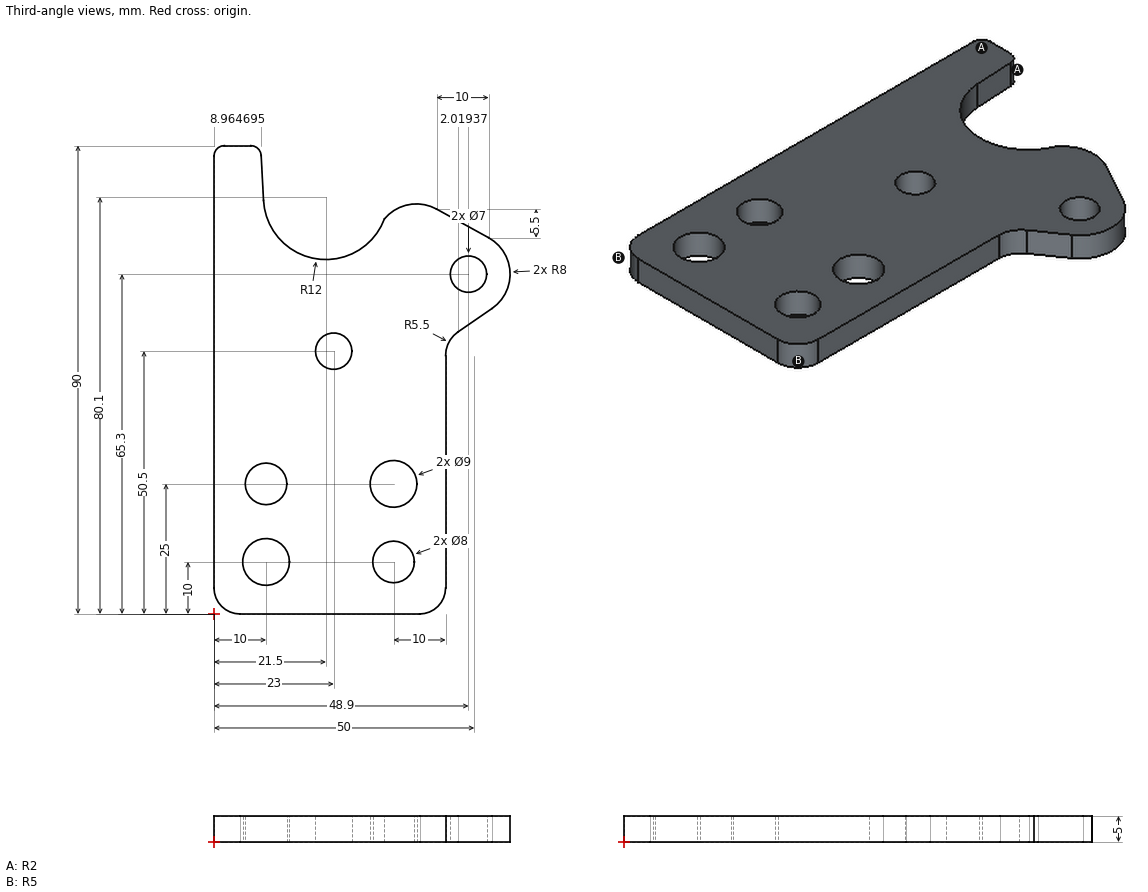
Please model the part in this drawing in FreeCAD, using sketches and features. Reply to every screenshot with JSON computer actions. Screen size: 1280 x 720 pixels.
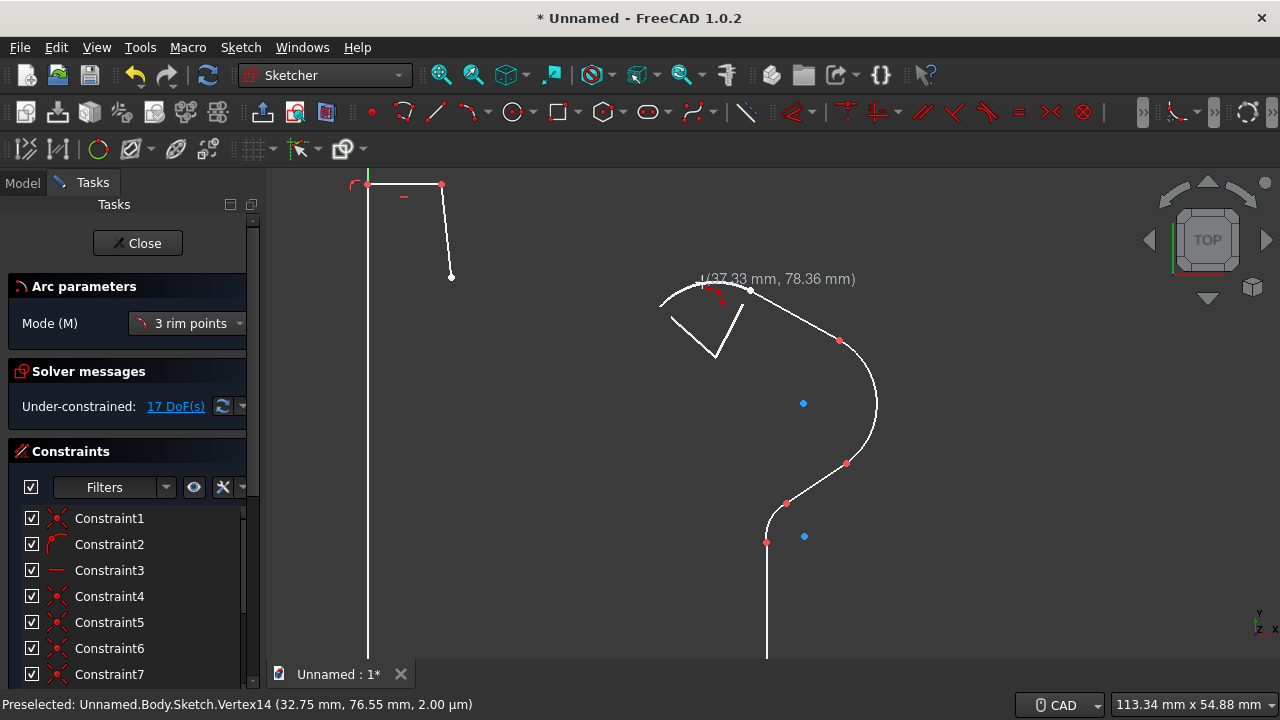
{"action": "left_click", "coordinate": [702, 281]}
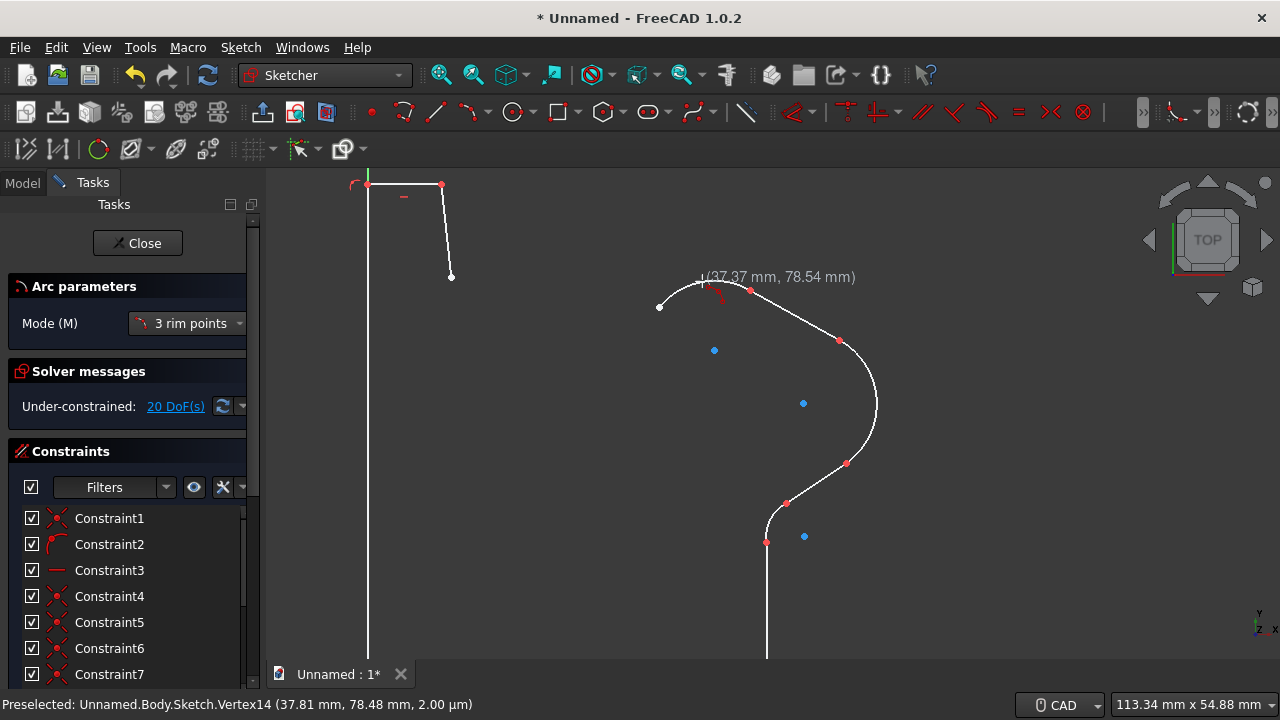
{"action": "left_click", "coordinate": [660, 307]}
{"action": "left_click", "coordinate": [451, 277]}
{"action": "left_click", "coordinate": [544, 374]}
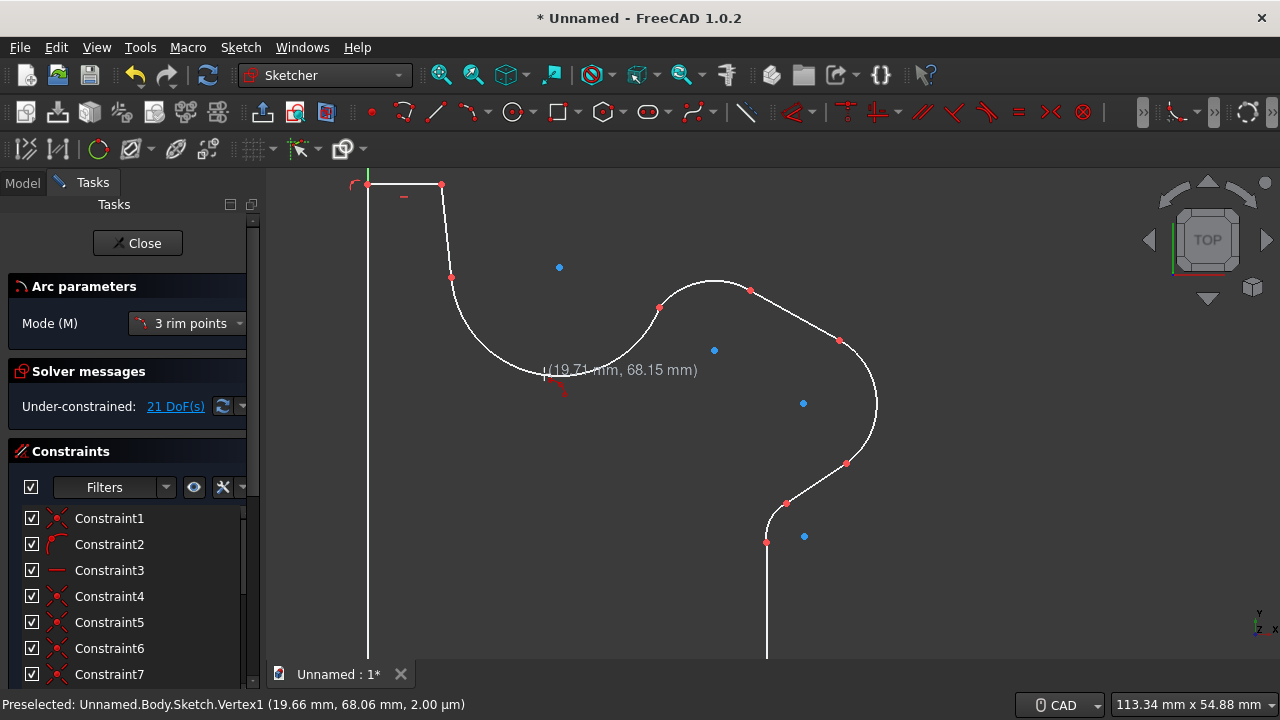
{"action": "key", "text": "g c"}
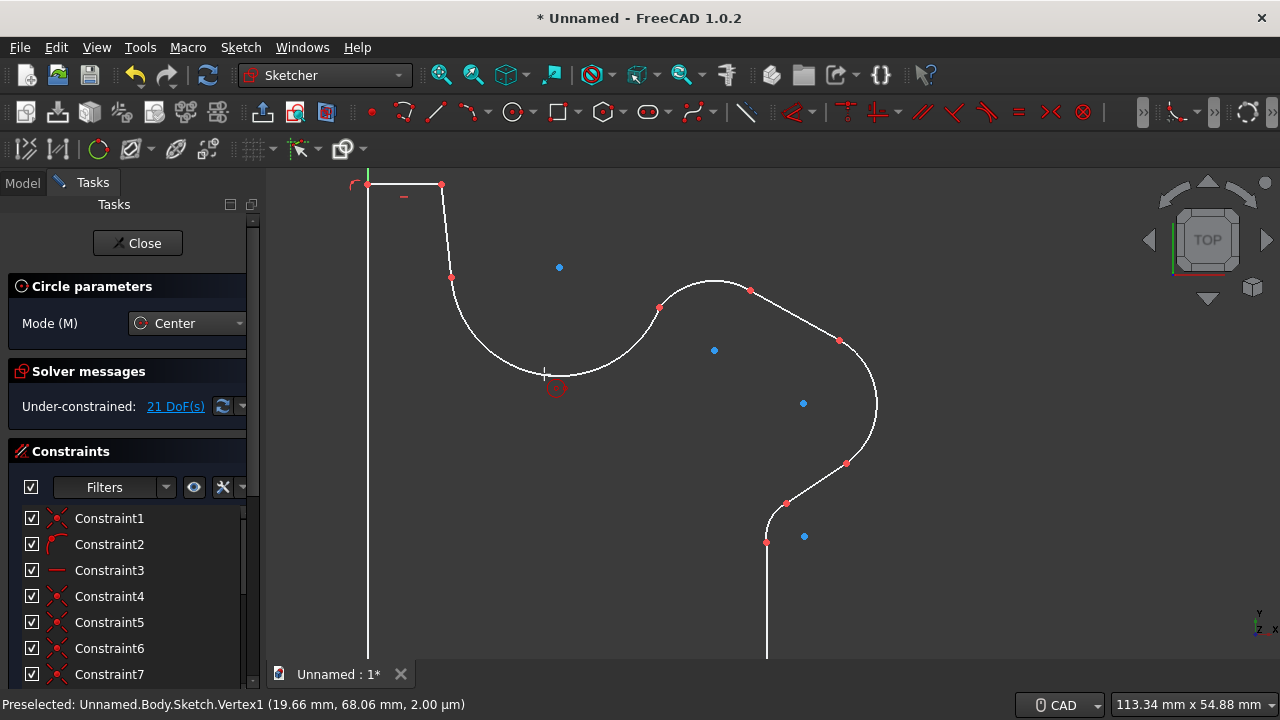
{"action": "scroll", "coordinate": [752, 315], "scroll_direction": "down", "scroll_amount": 5}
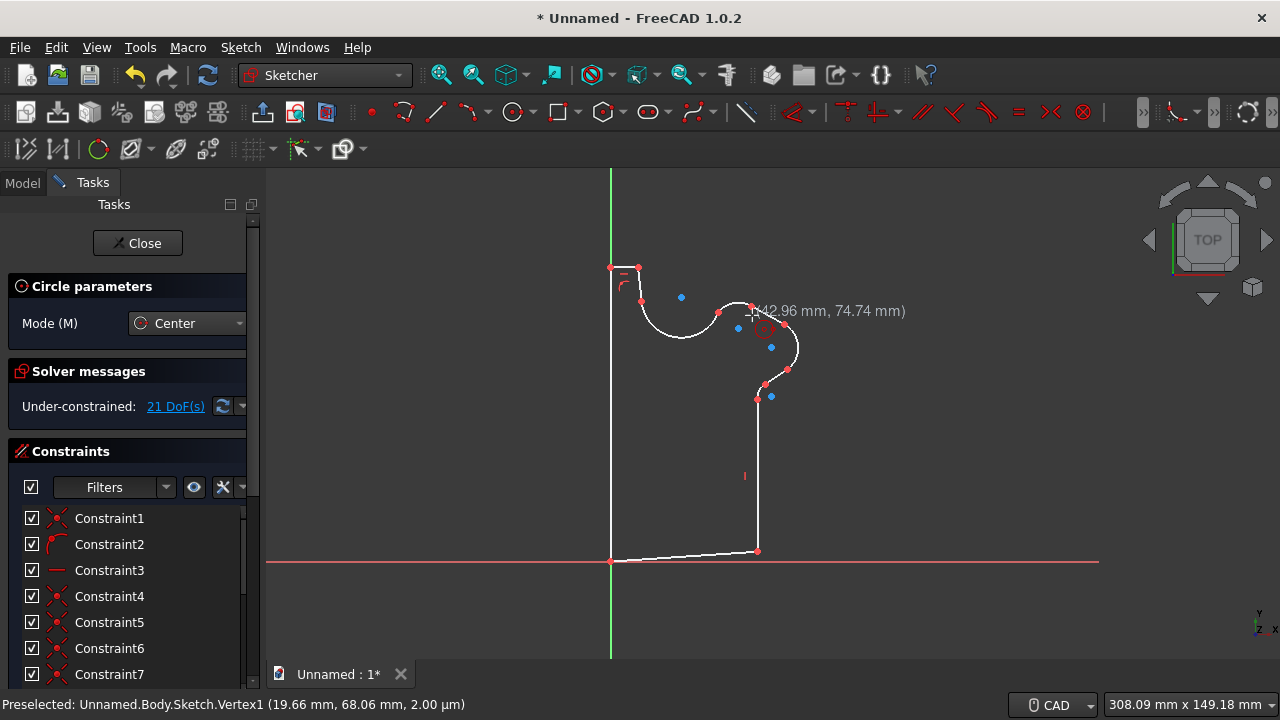
{"action": "scroll", "coordinate": [724, 529], "scroll_direction": "up", "scroll_amount": 3}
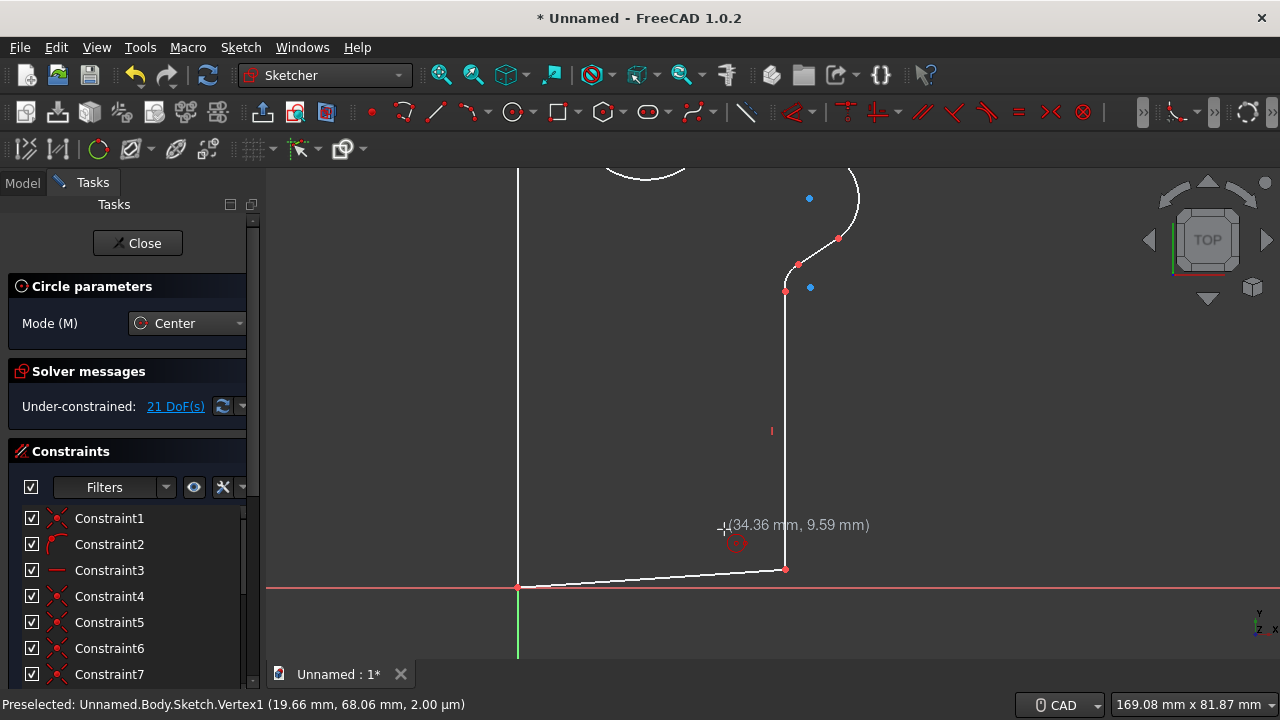
{"action": "left_click", "coordinate": [724, 528]}
{"action": "left_click", "coordinate": [741, 511]}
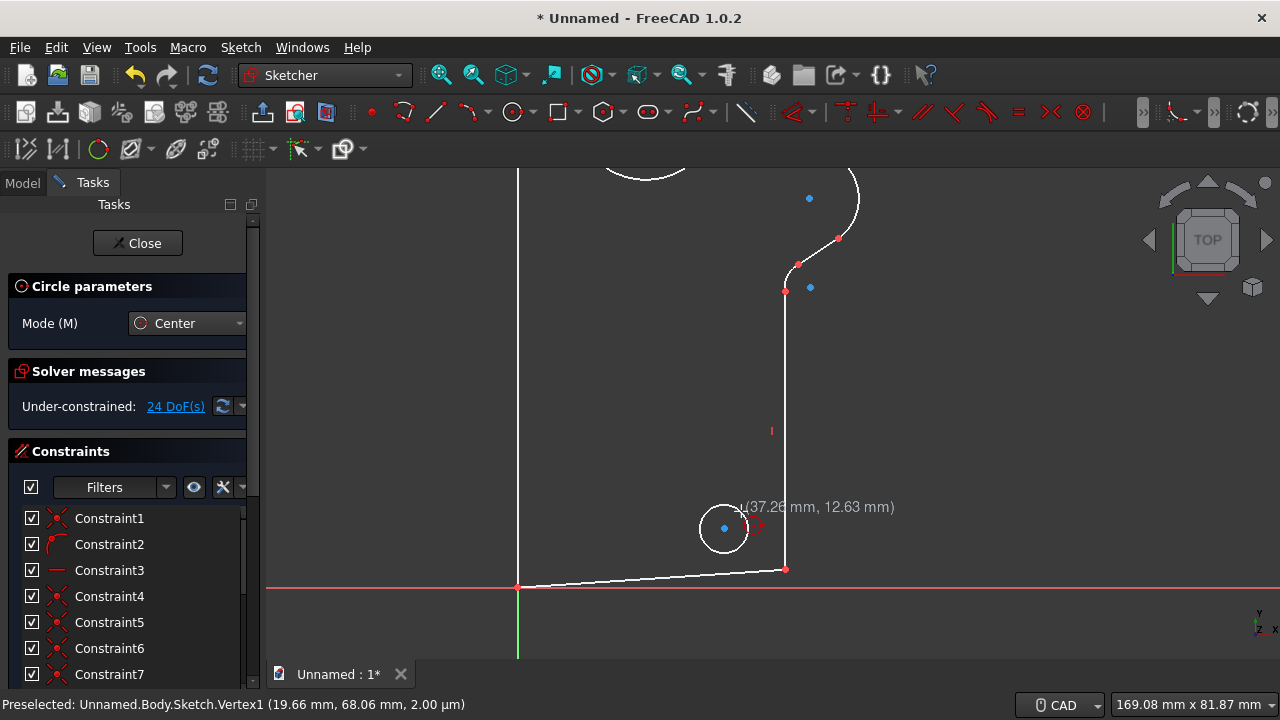
{"action": "left_click", "coordinate": [724, 438]}
{"action": "left_click", "coordinate": [744, 419]}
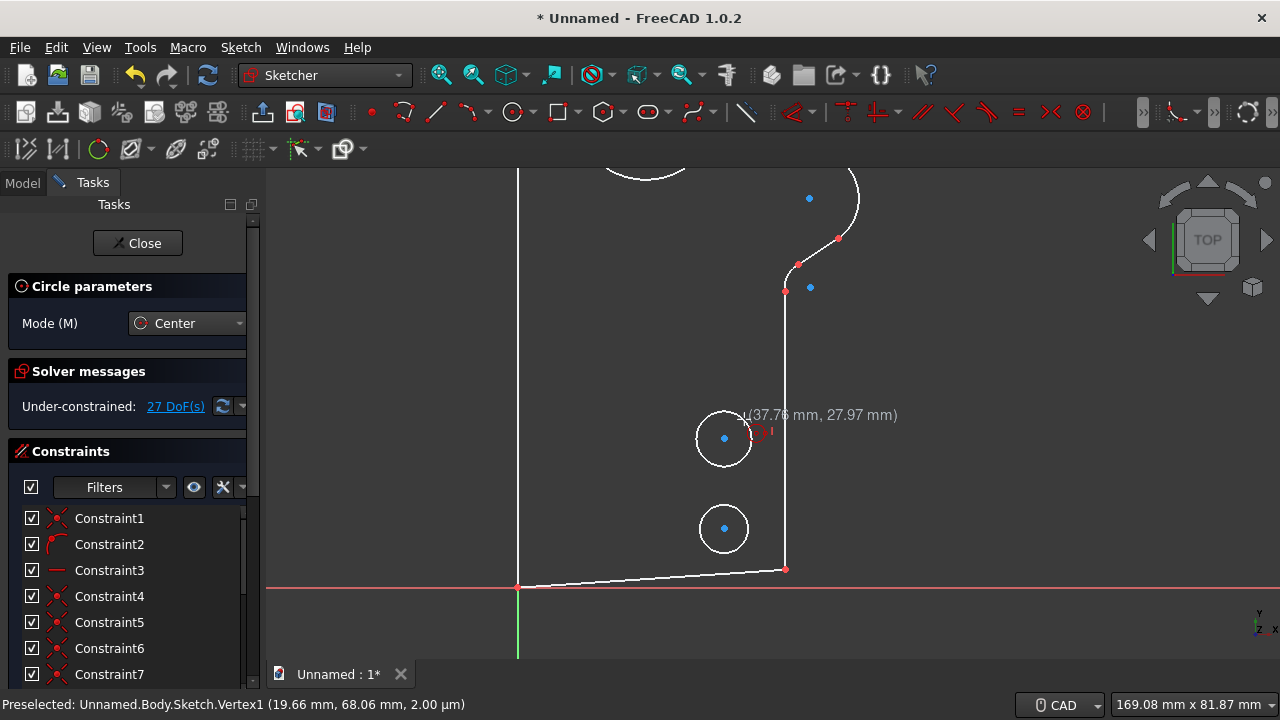
{"action": "left_click", "coordinate": [578, 528]}
{"action": "left_click", "coordinate": [597, 509]}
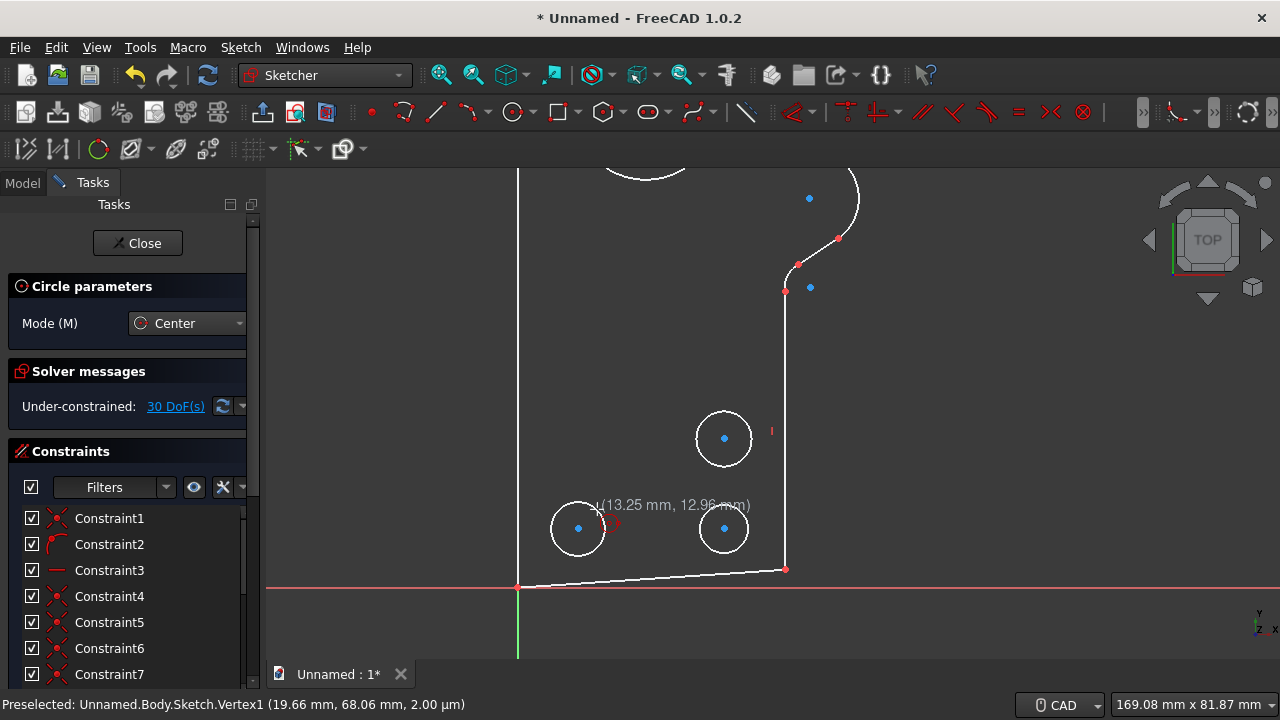
{"action": "left_click", "coordinate": [578, 438]}
{"action": "left_click", "coordinate": [594, 421]}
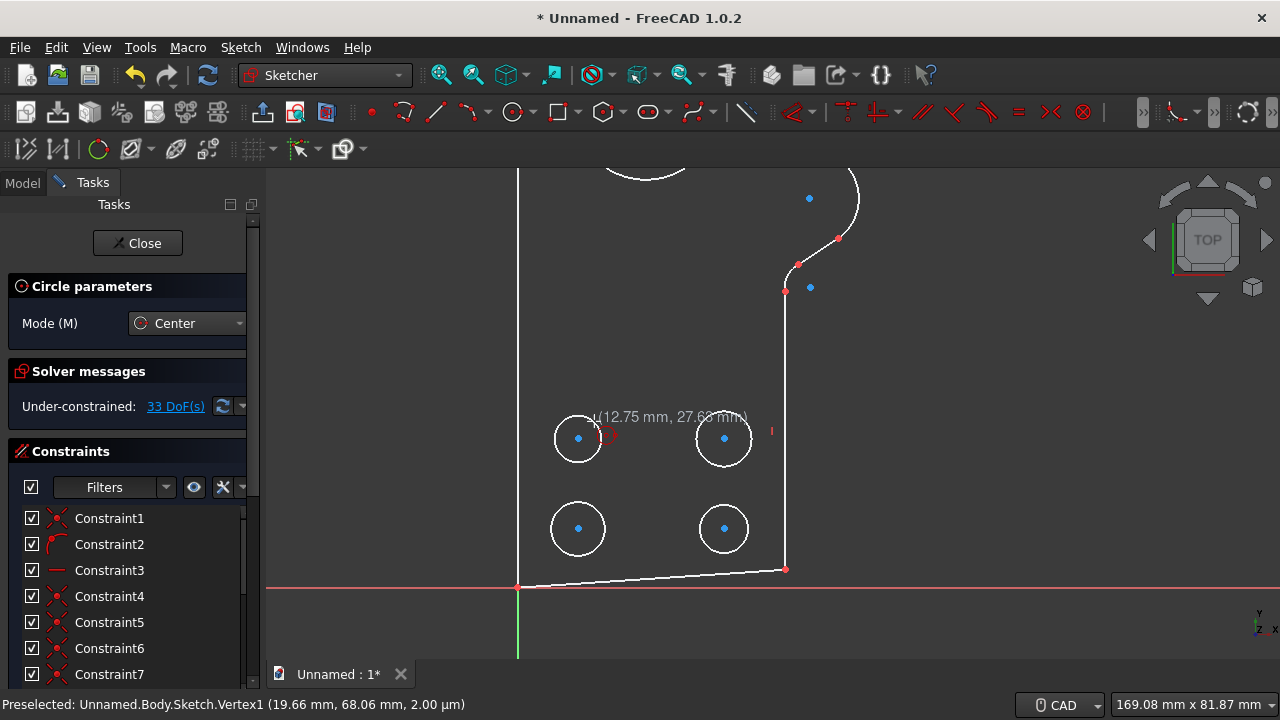
{"action": "left_click", "coordinate": [811, 196]}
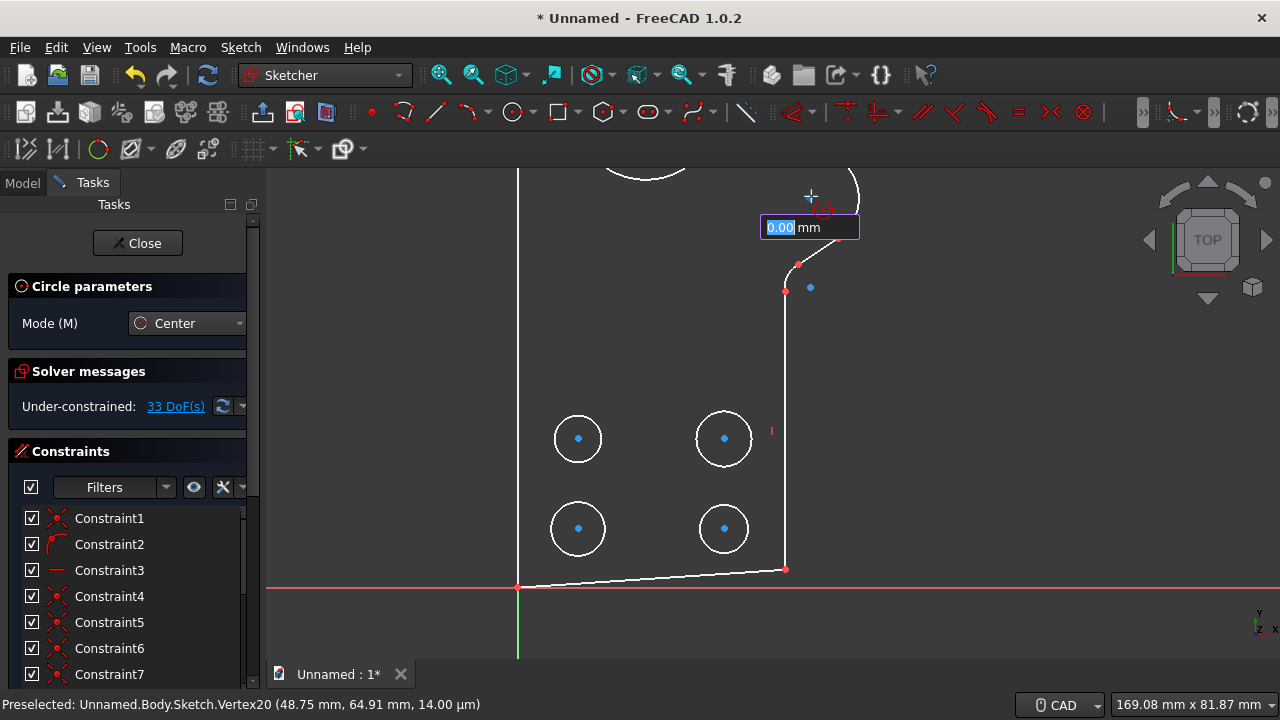
{"action": "scroll", "coordinate": [724, 530], "scroll_direction": "down", "scroll_amount": 3}